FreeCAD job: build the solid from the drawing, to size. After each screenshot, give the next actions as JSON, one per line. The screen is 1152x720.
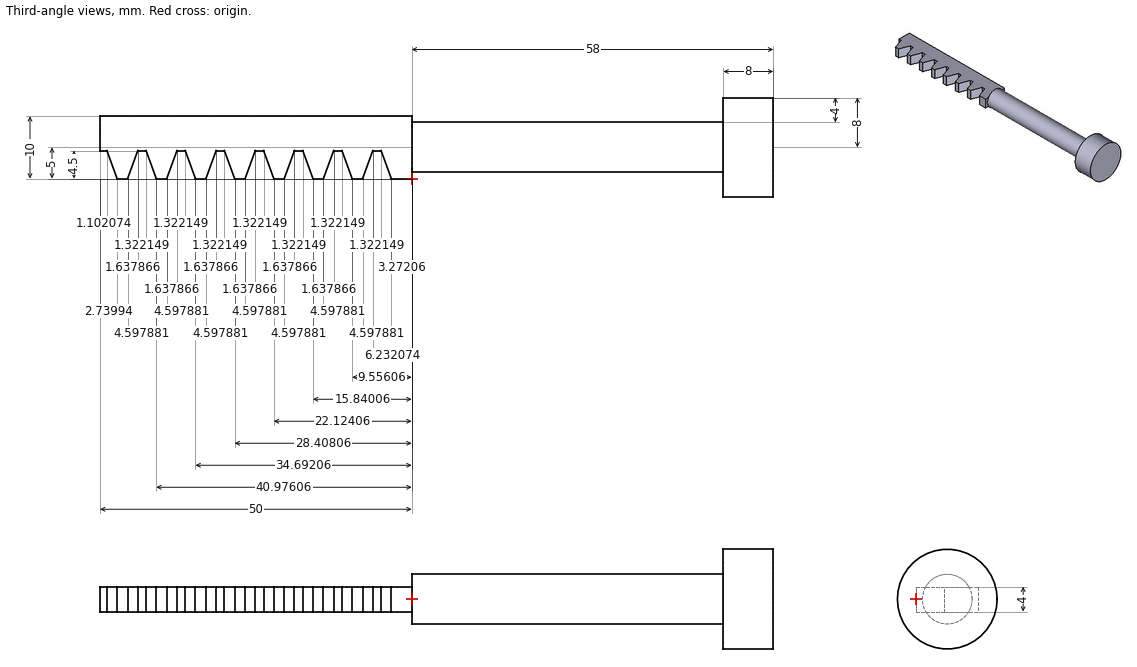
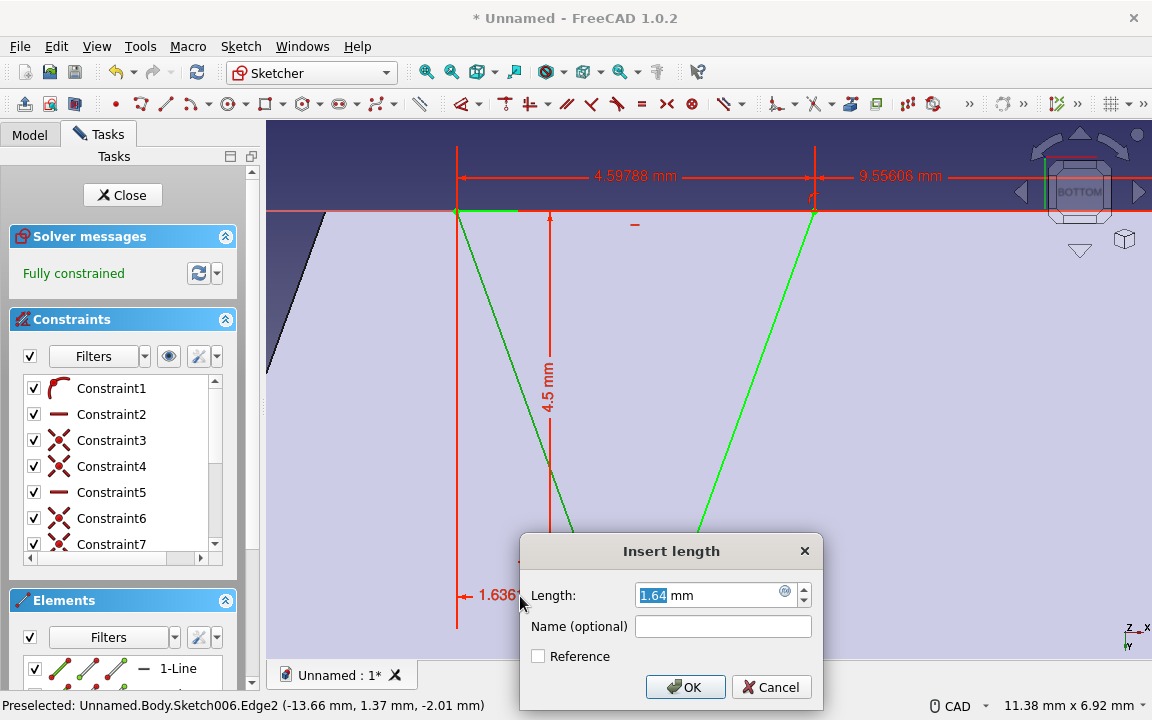
{"action": "type", "text": "1.637866"}
{"action": "key", "text": "Return"}
{"action": "key", "text": "Escape"}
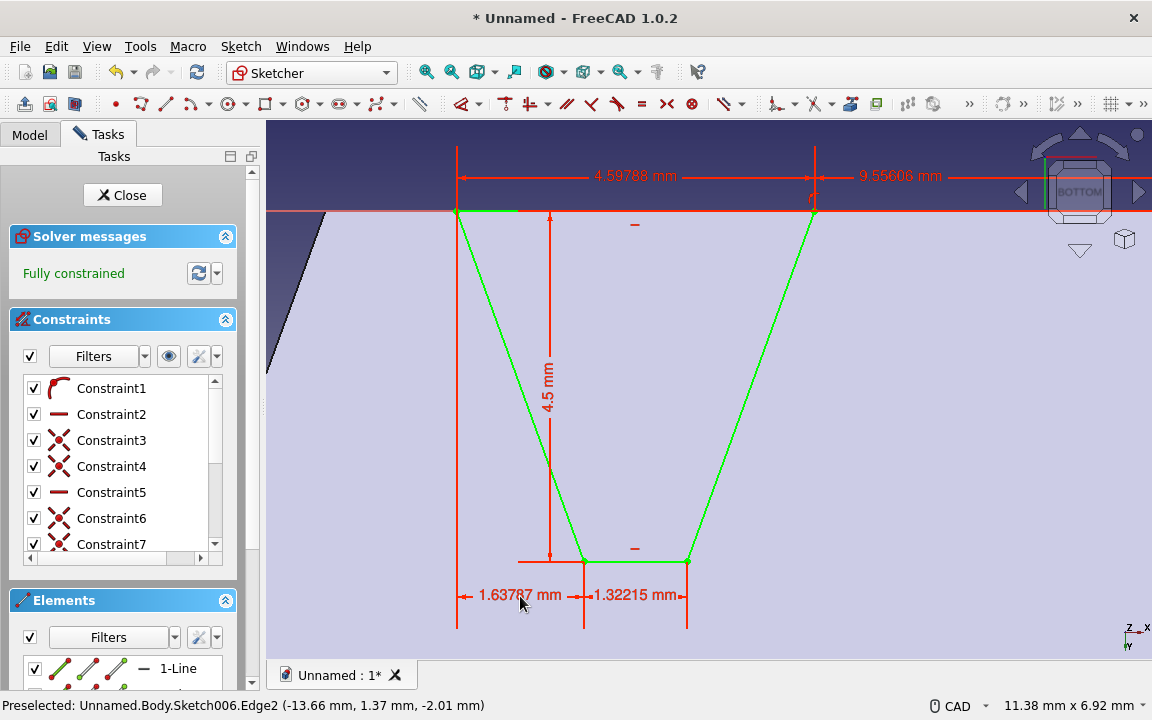
{"action": "left_click", "coordinate": [123, 195]}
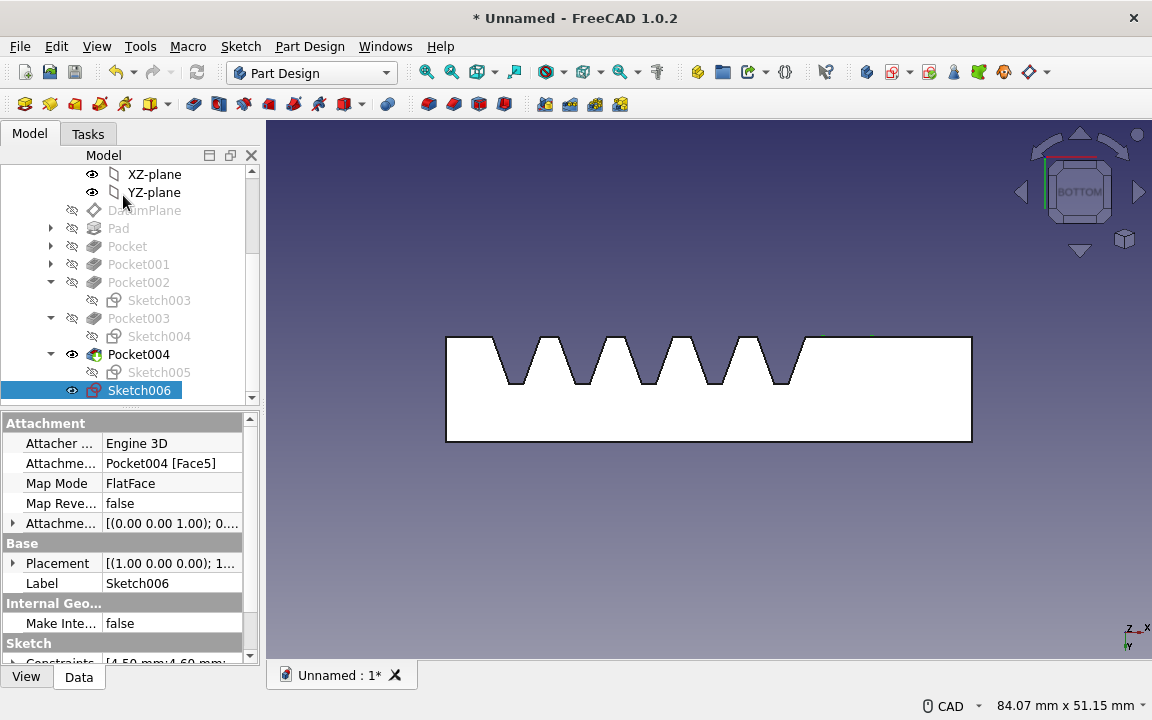
{"action": "left_click", "coordinate": [194, 104]}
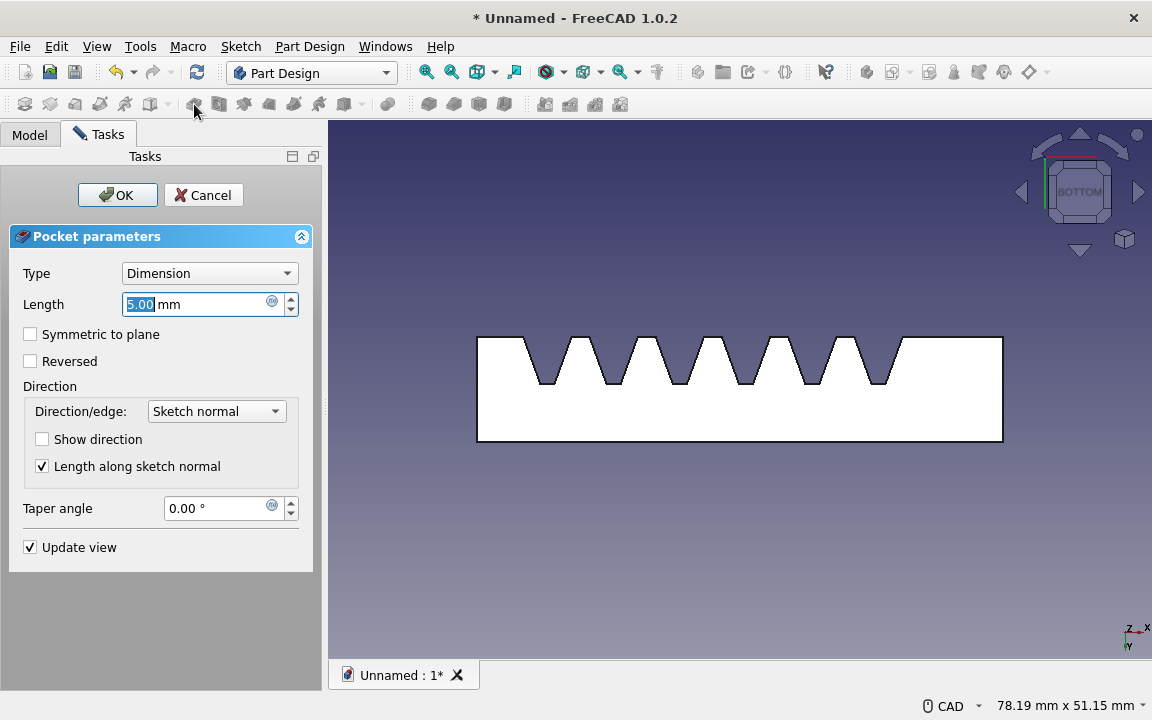
{"action": "left_click", "coordinate": [210, 274]}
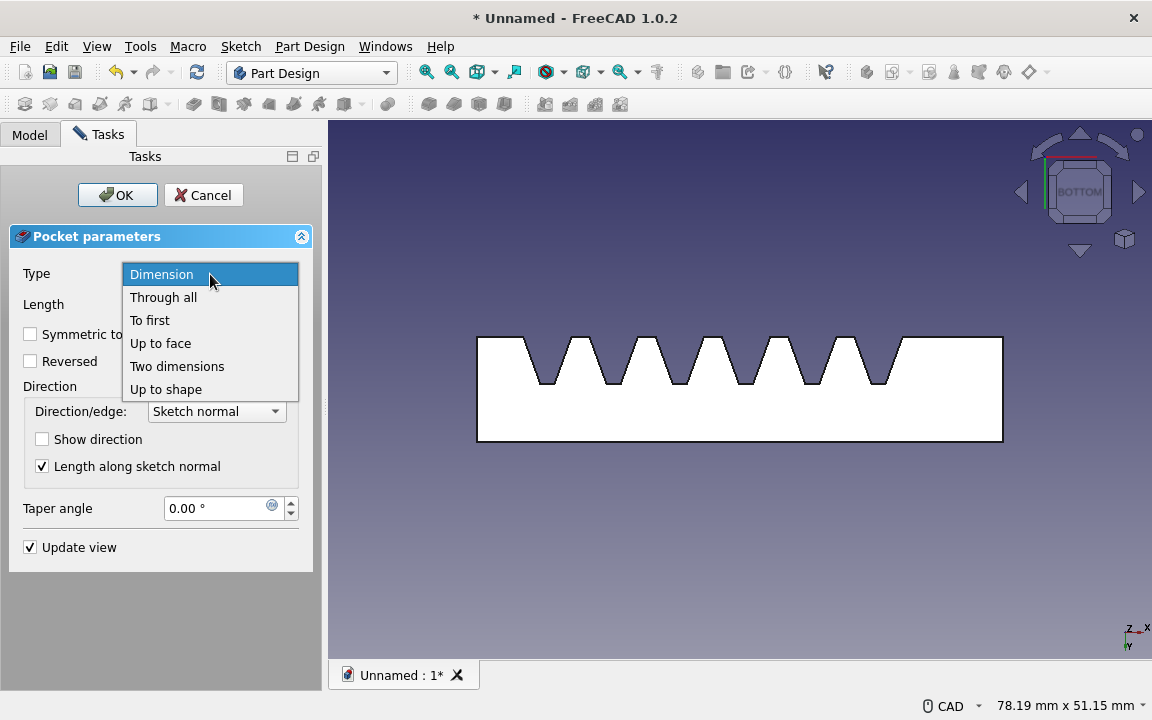
{"action": "left_click", "coordinate": [208, 298]}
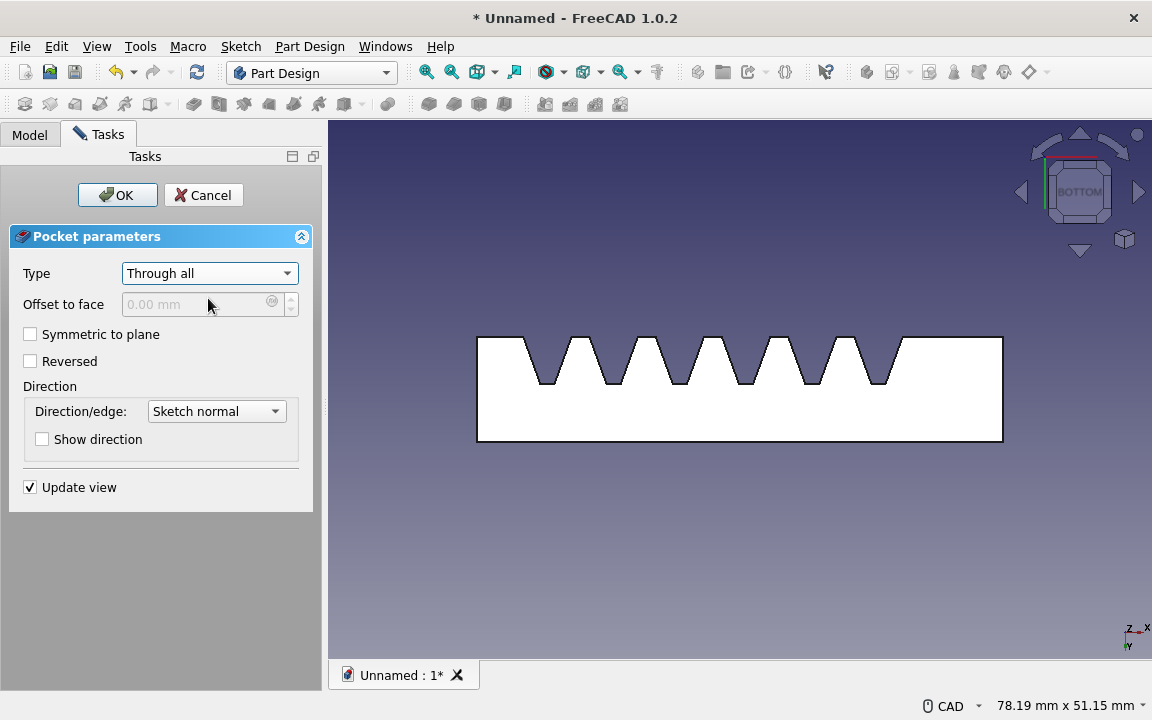
{"action": "left_click", "coordinate": [118, 195]}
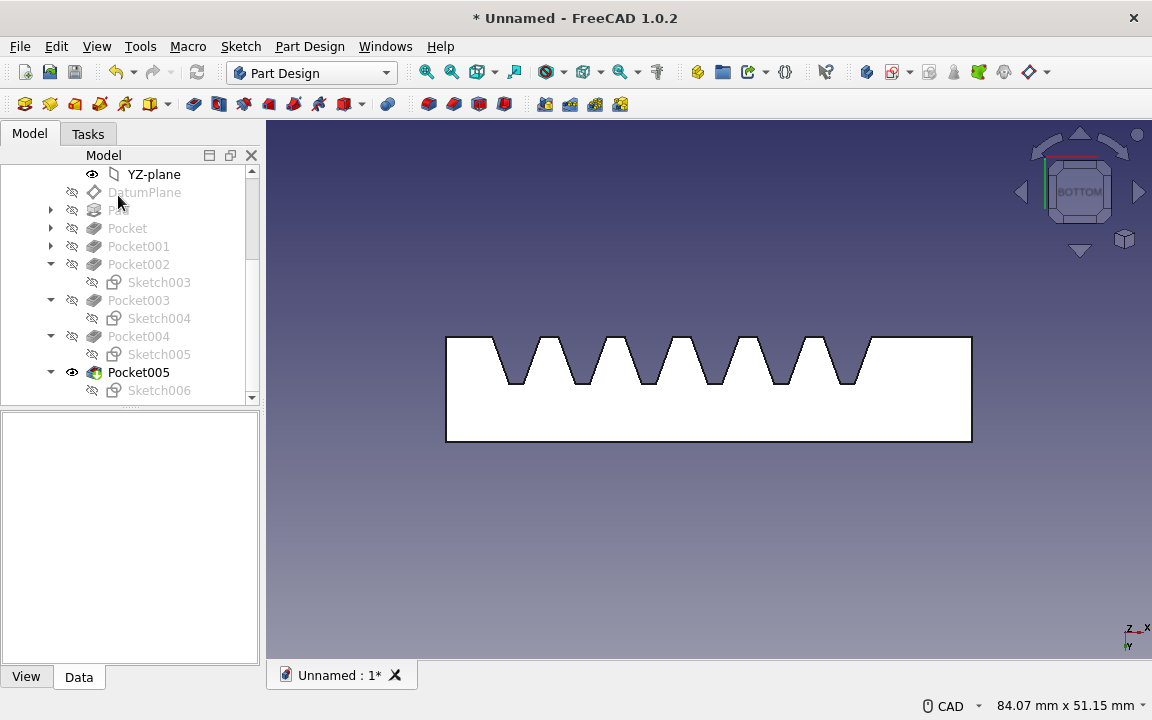
{"action": "left_click", "coordinate": [935, 404]}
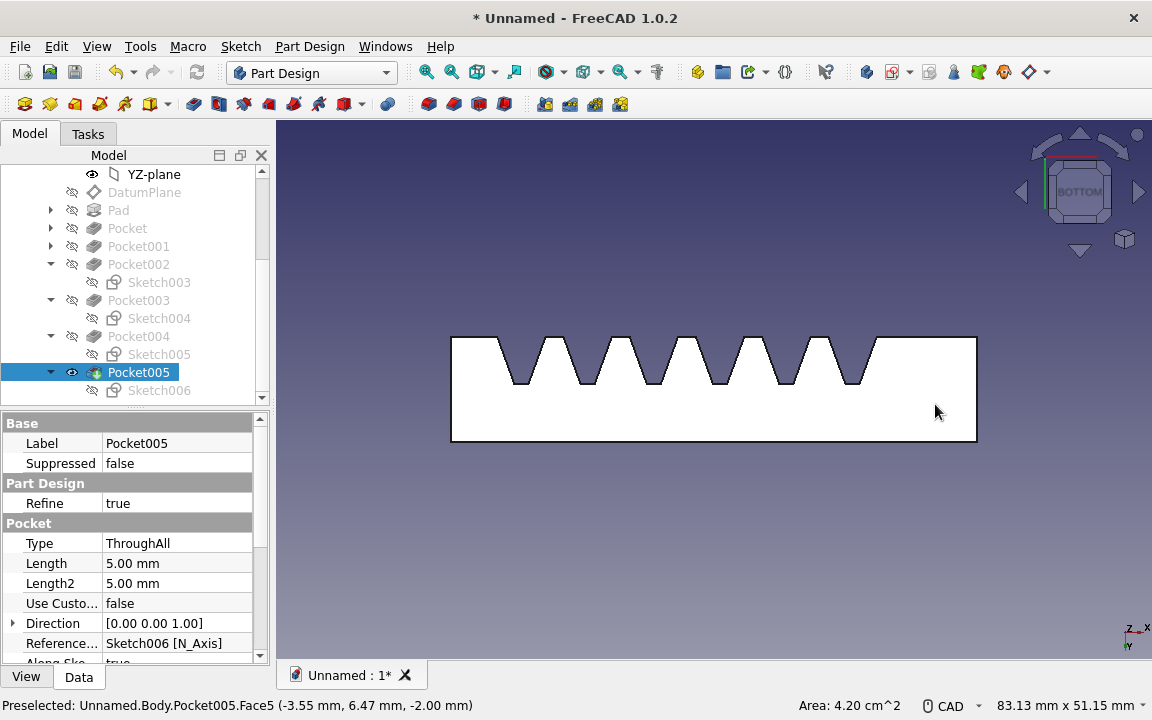
{"action": "left_click", "coordinate": [892, 72]}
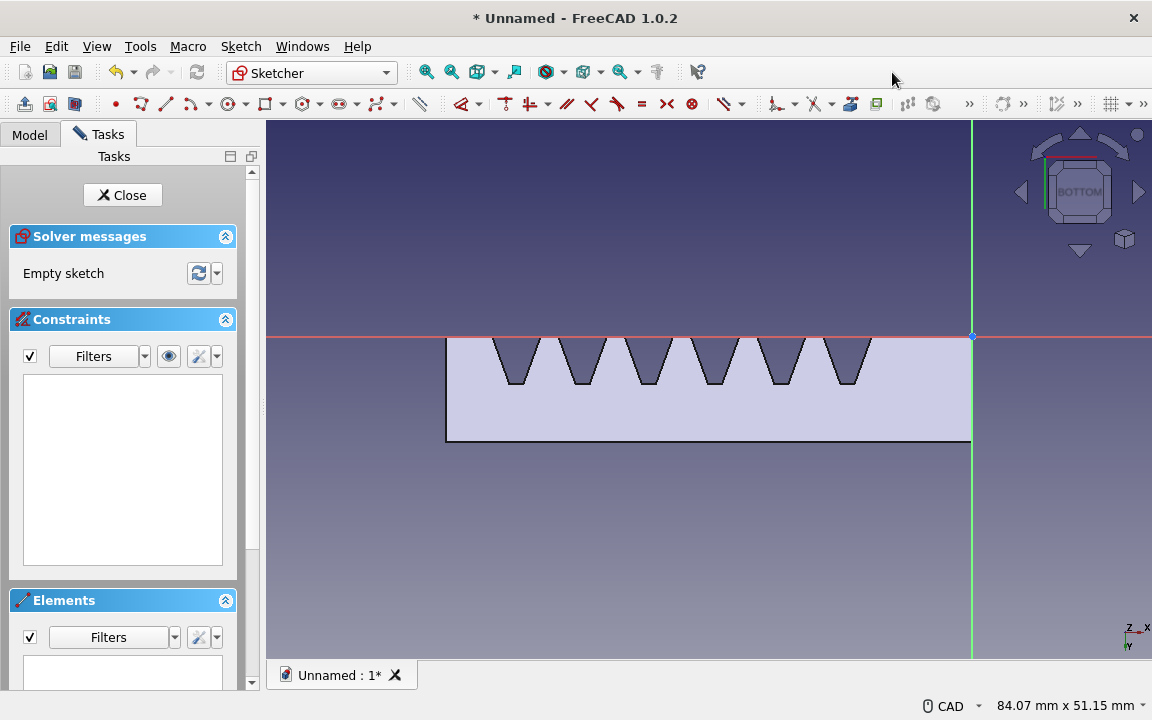
{"action": "scroll", "coordinate": [987, 355], "scroll_direction": "up", "scroll_amount": 9}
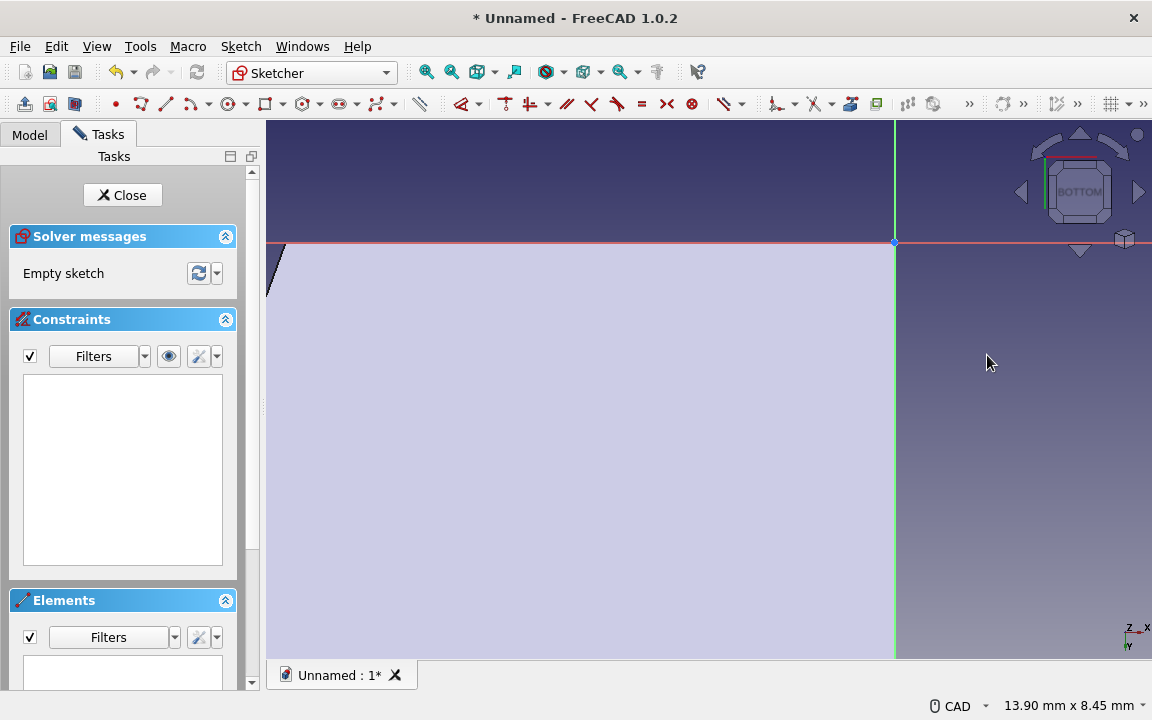
{"action": "left_click", "coordinate": [141, 104]}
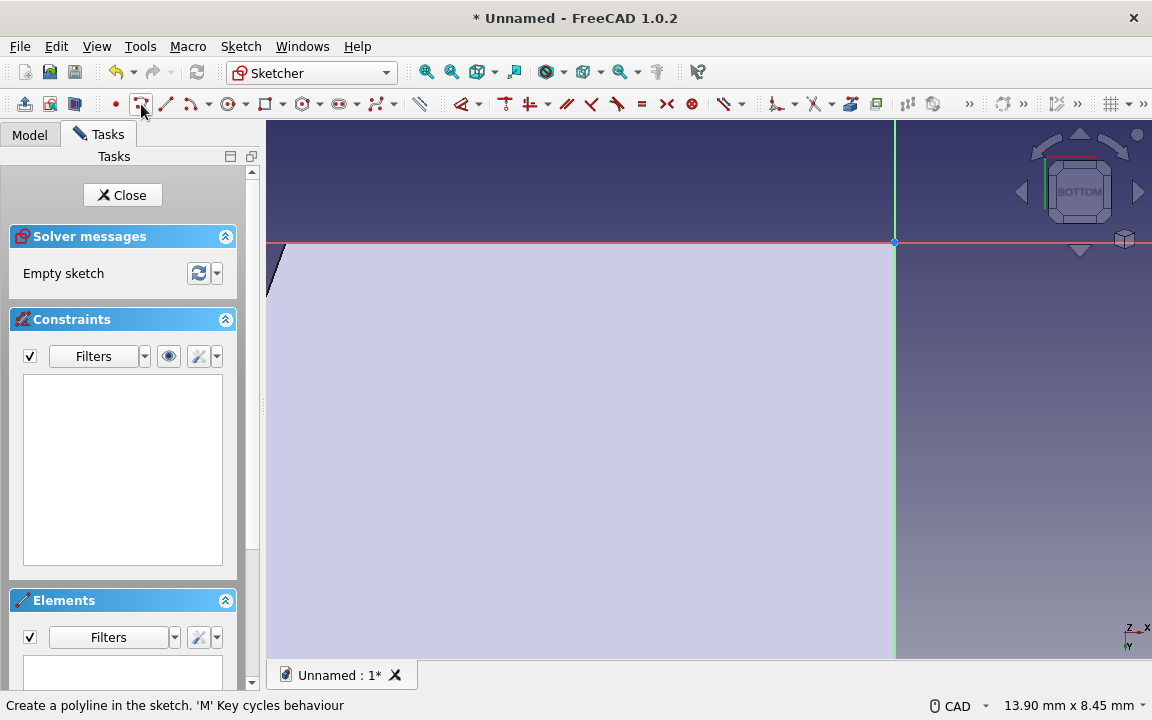
{"action": "left_click", "coordinate": [686, 243]}
{"action": "left_click", "coordinate": [393, 252]}
{"action": "left_click", "coordinate": [498, 530]}
{"action": "left_click", "coordinate": [582, 530]}
{"action": "left_click", "coordinate": [686, 243]}
{"action": "key", "text": "Escape"}
{"action": "key", "text": "Escape"}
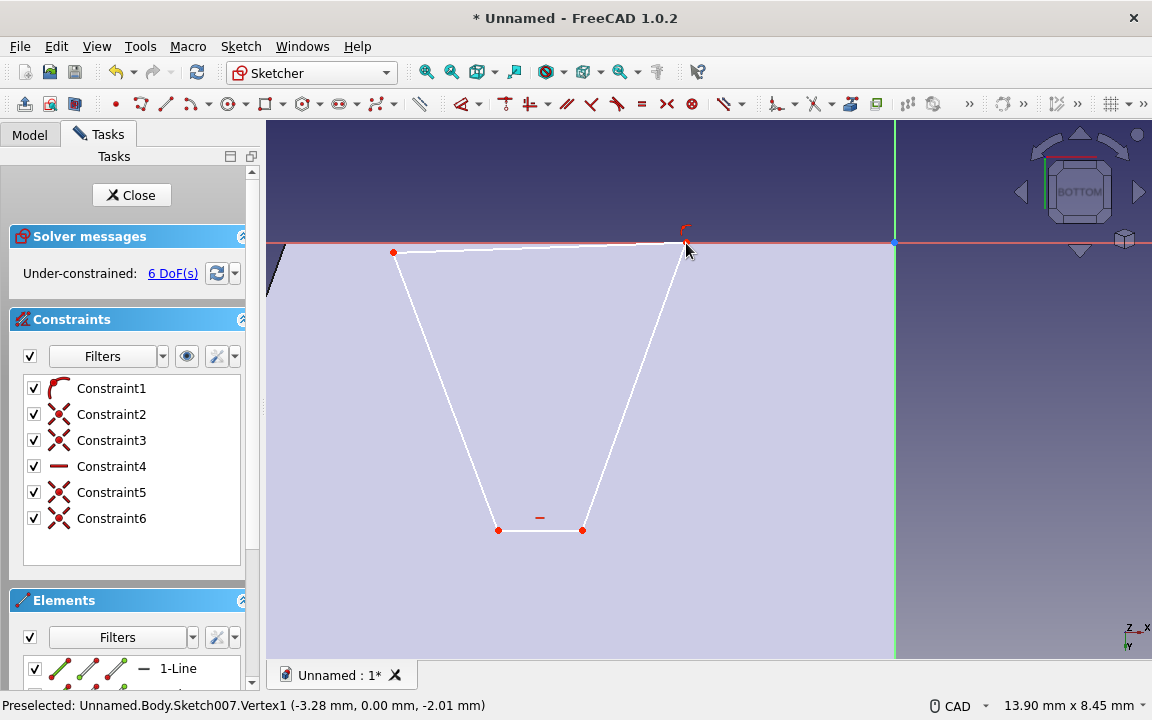
{"action": "left_click", "coordinate": [598, 246]}